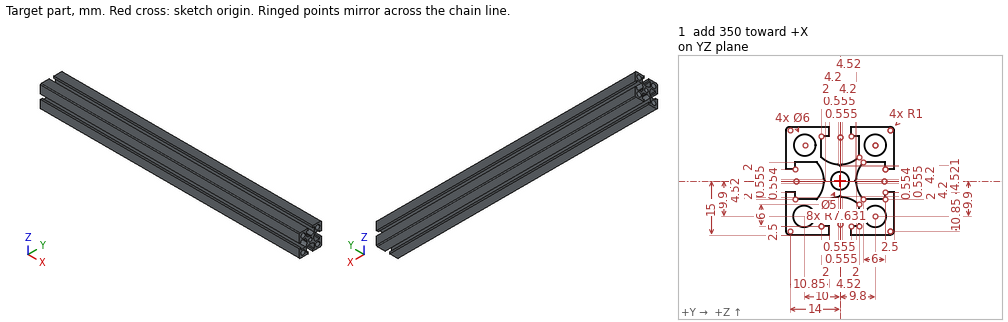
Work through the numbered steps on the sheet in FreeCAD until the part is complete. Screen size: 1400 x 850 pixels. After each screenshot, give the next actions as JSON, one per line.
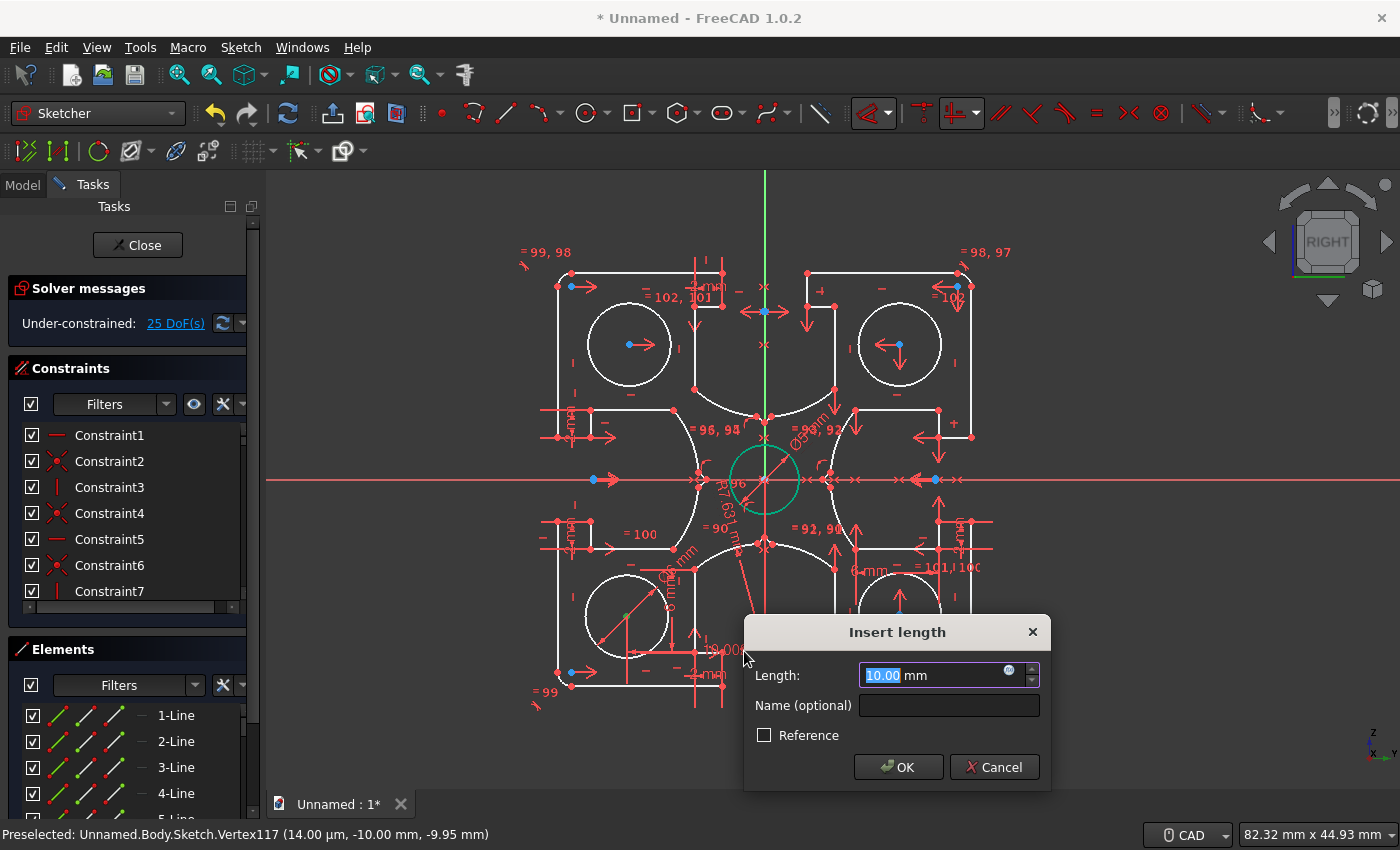
{"action": "type", "text": "10"}
{"action": "key", "text": "Return"}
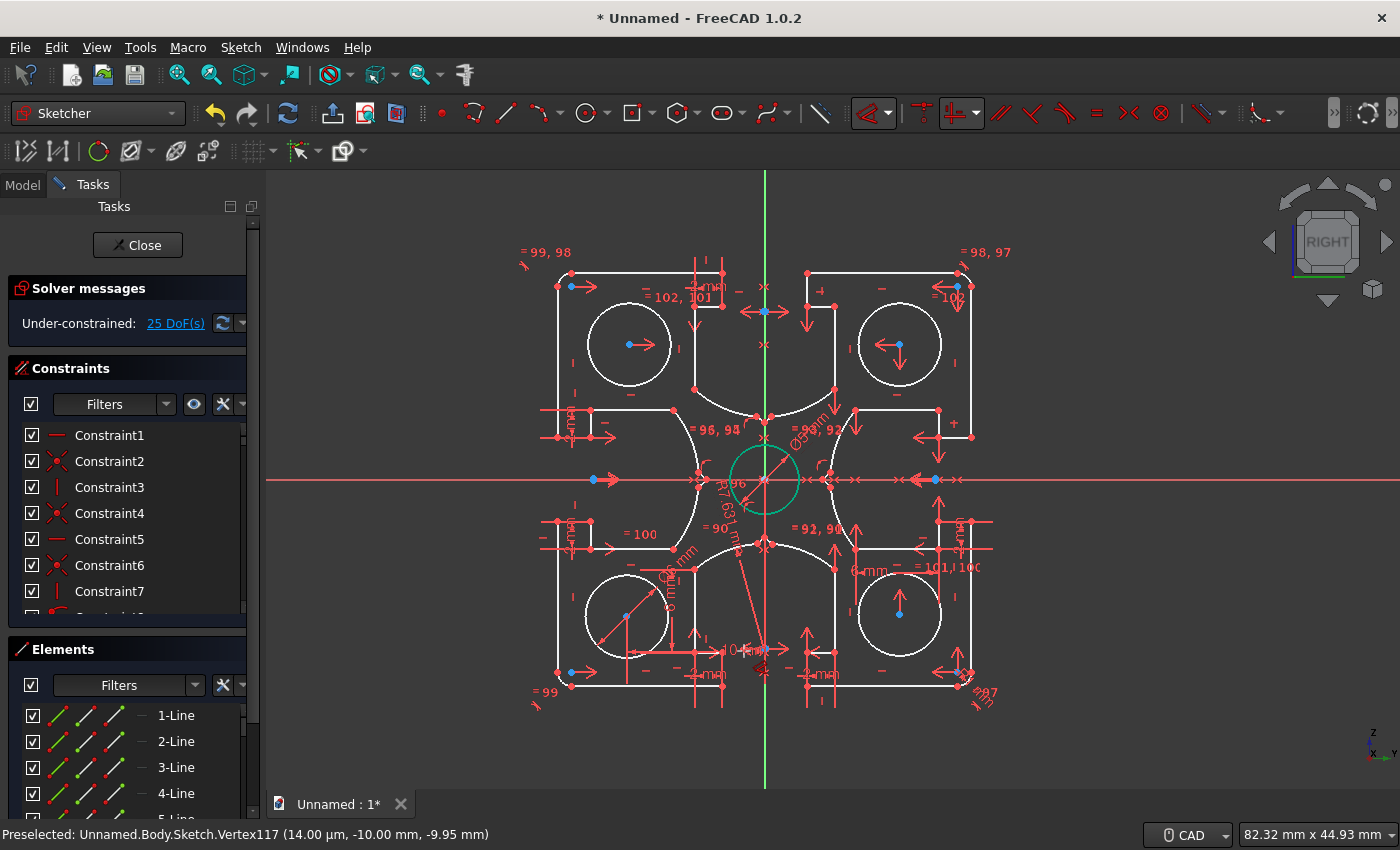
{"action": "scroll", "coordinate": [722, 676], "scroll_direction": "up", "scroll_amount": 2}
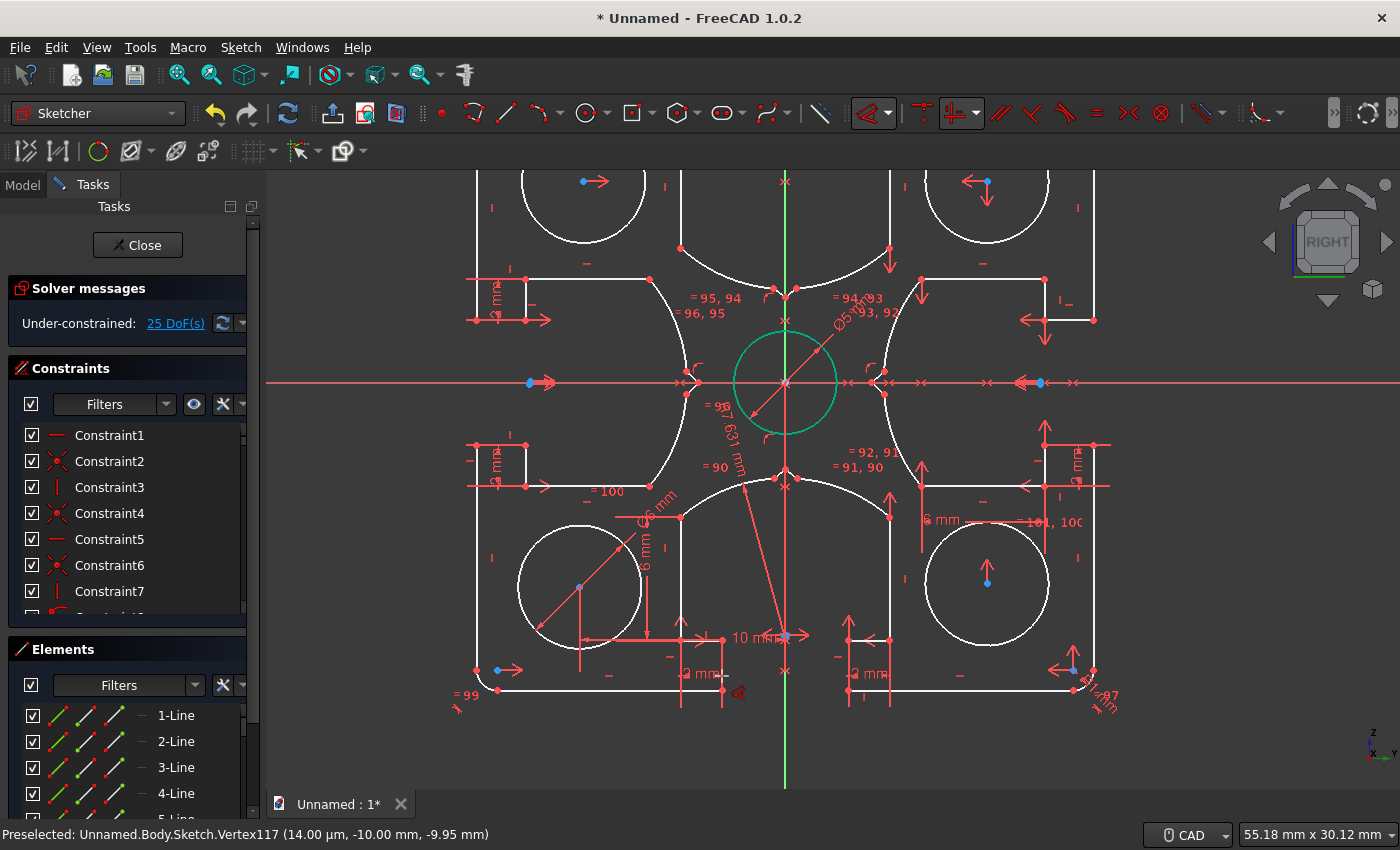
{"action": "left_click", "coordinate": [722, 676]}
{"action": "left_click", "coordinate": [664, 648]}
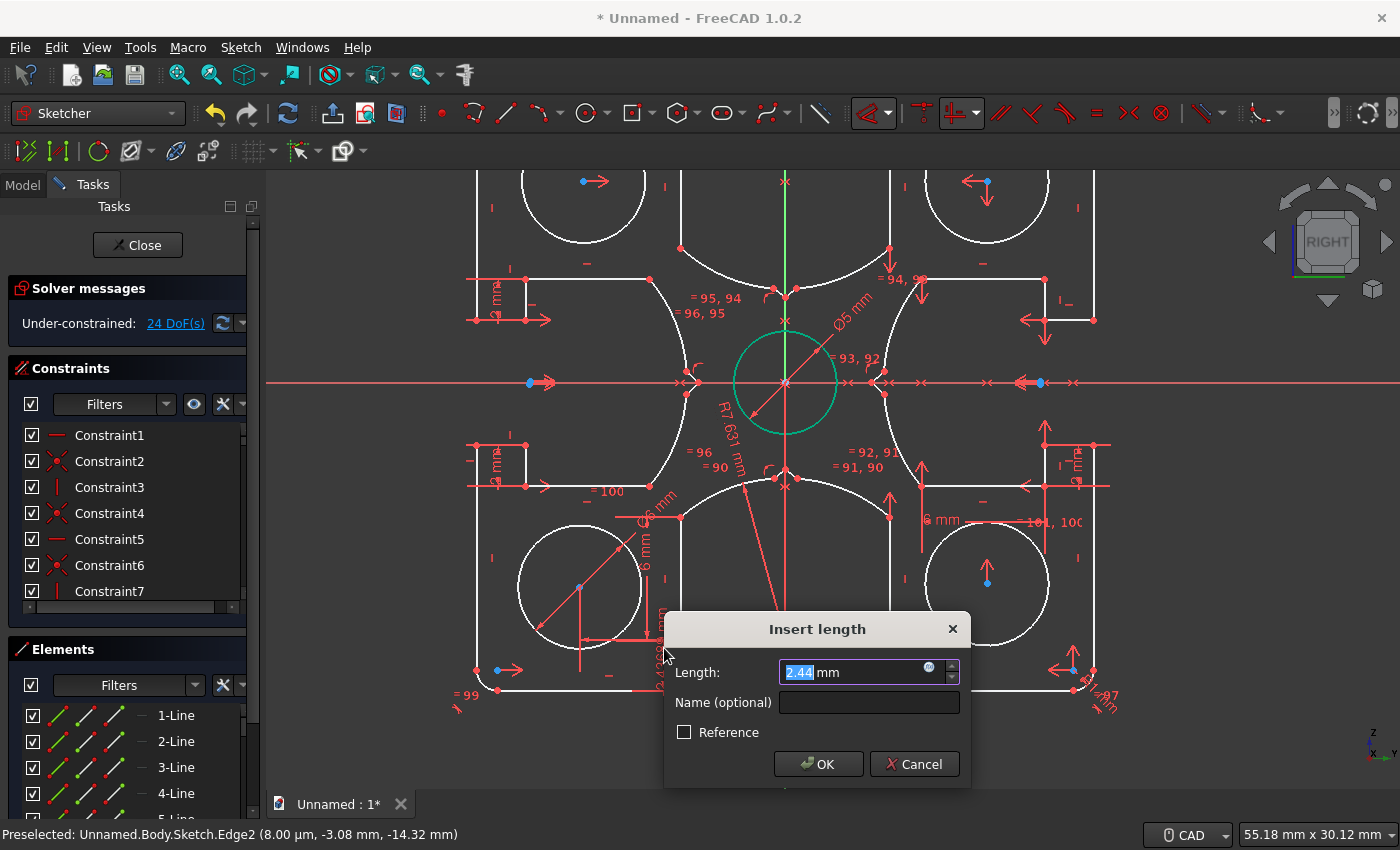
{"action": "type", "text": "2.5"}
{"action": "key", "text": "Return"}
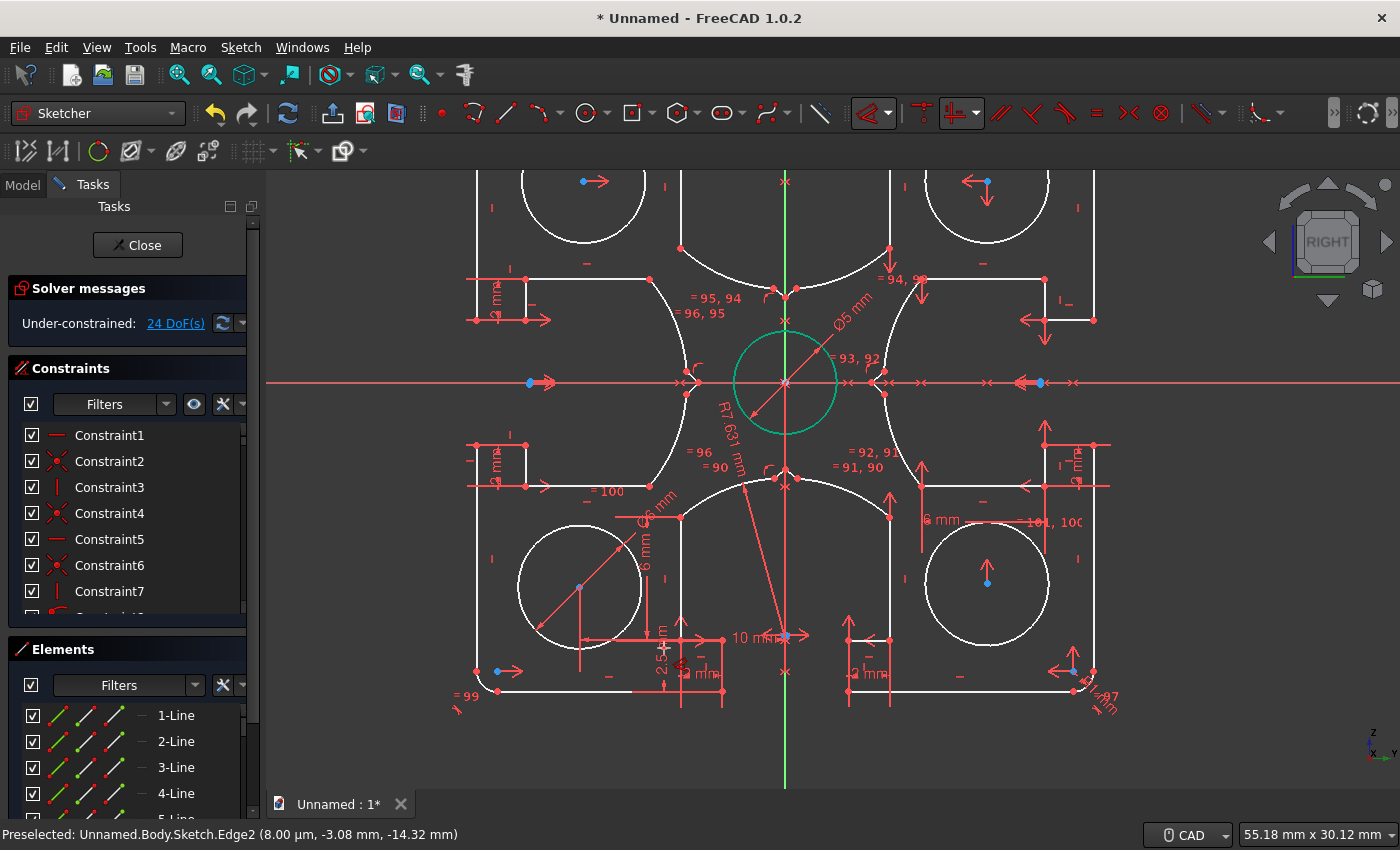
{"action": "left_click", "coordinate": [1079, 445]}
{"action": "left_click", "coordinate": [1069, 411]}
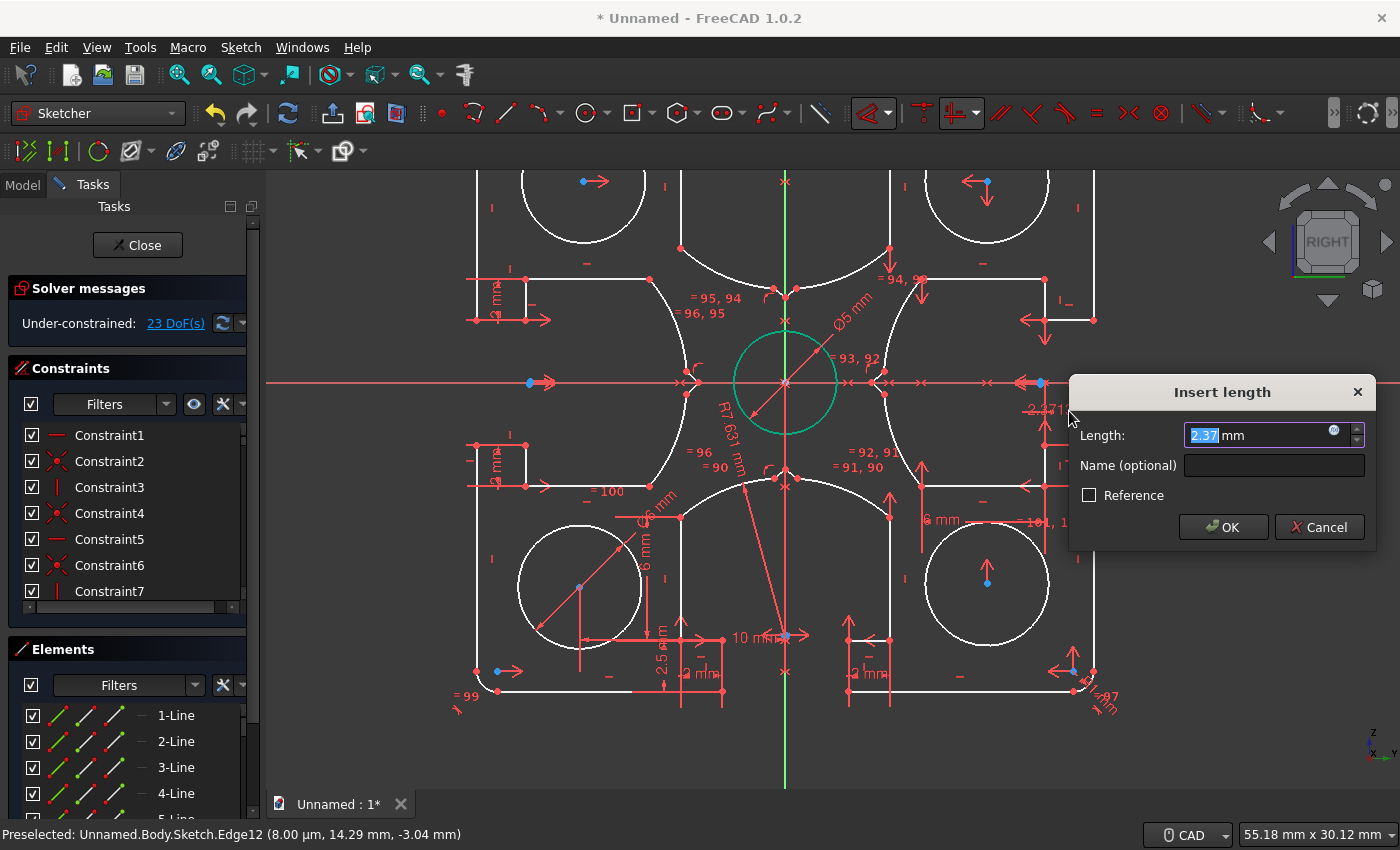
{"action": "type", "text": "2.5"}
{"action": "key", "text": "Return"}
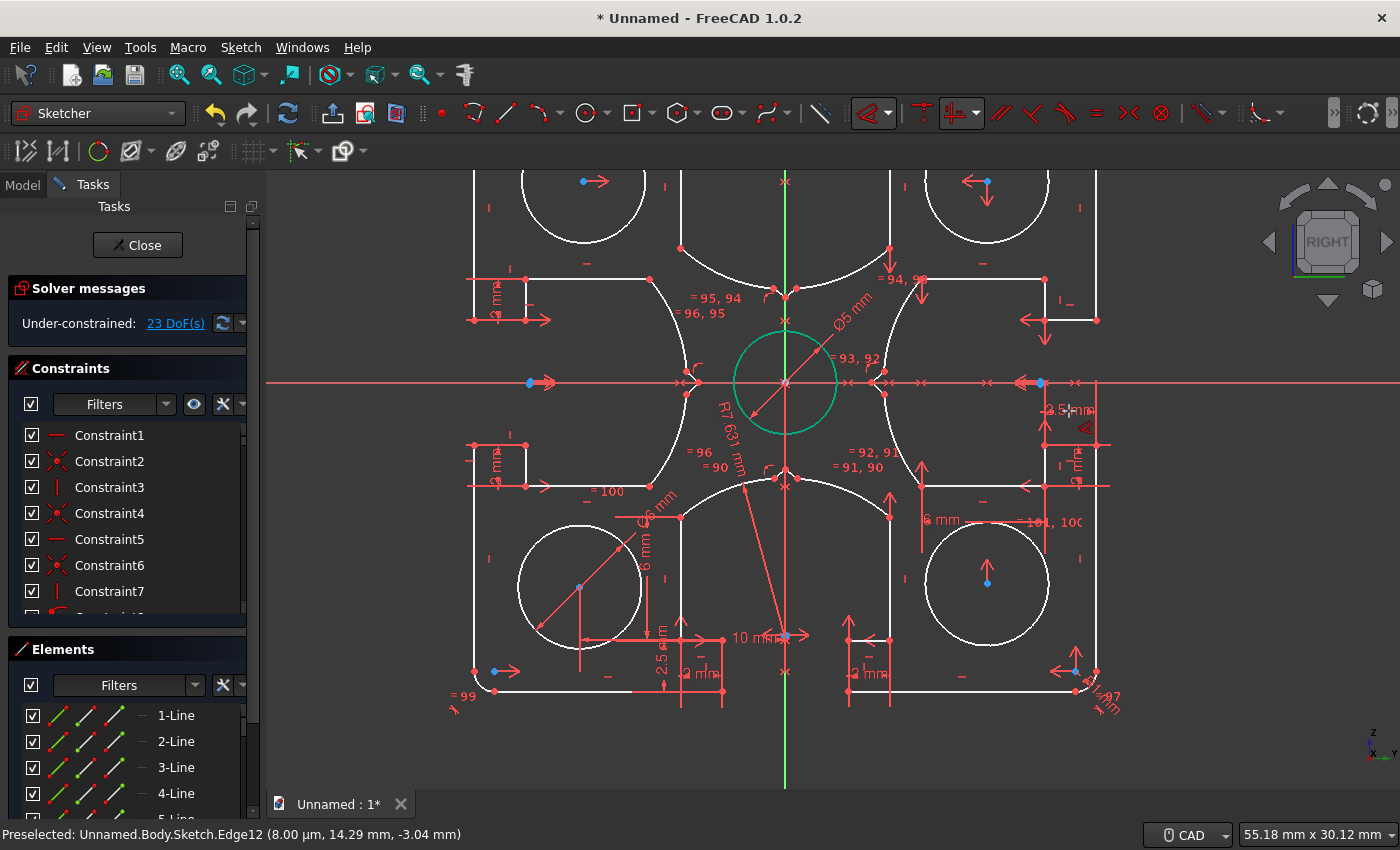
{"action": "left_click", "coordinate": [495, 692]}
{"action": "left_click", "coordinate": [640, 726]}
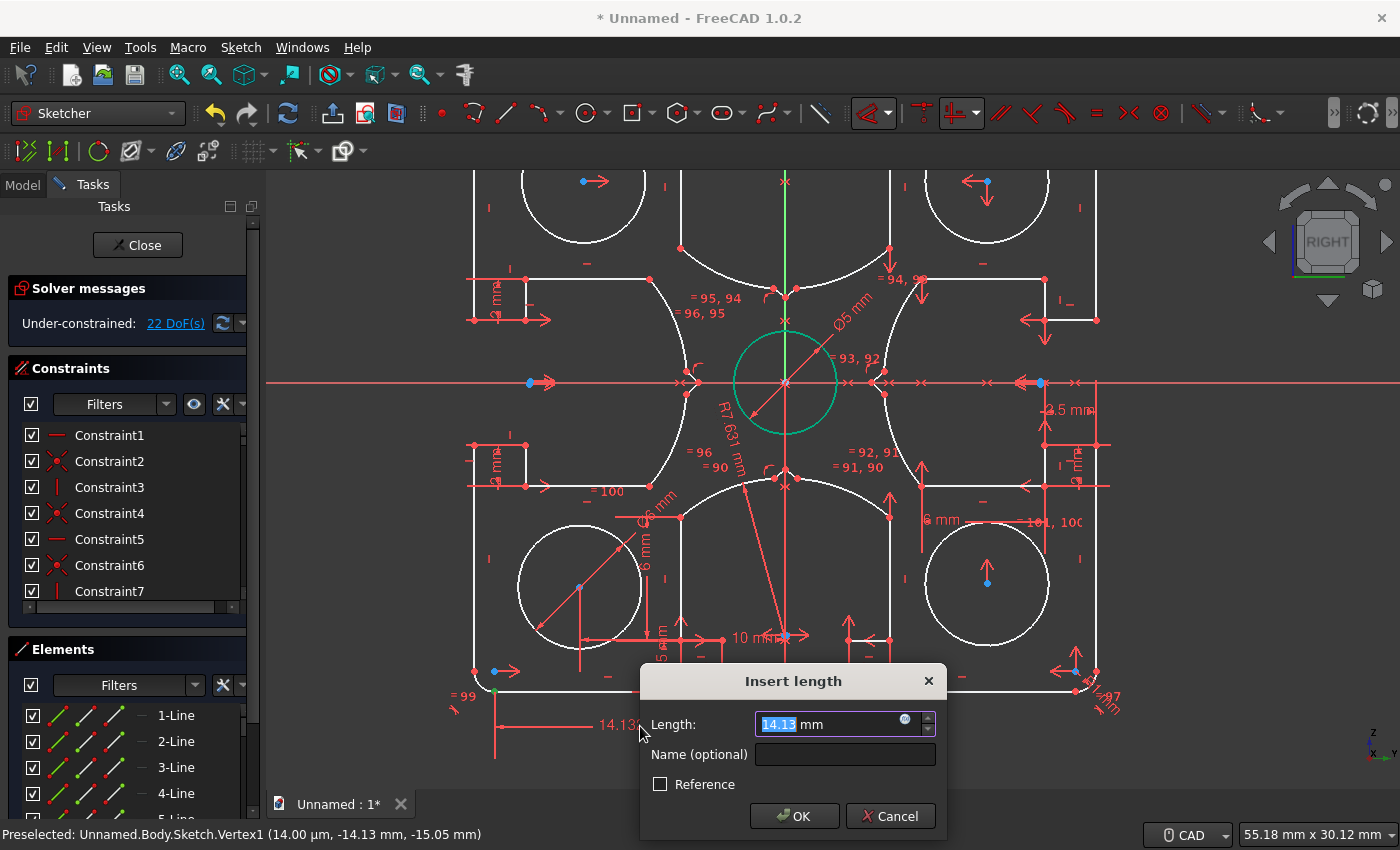
{"action": "type", "text": "14"}
{"action": "key", "text": "Return"}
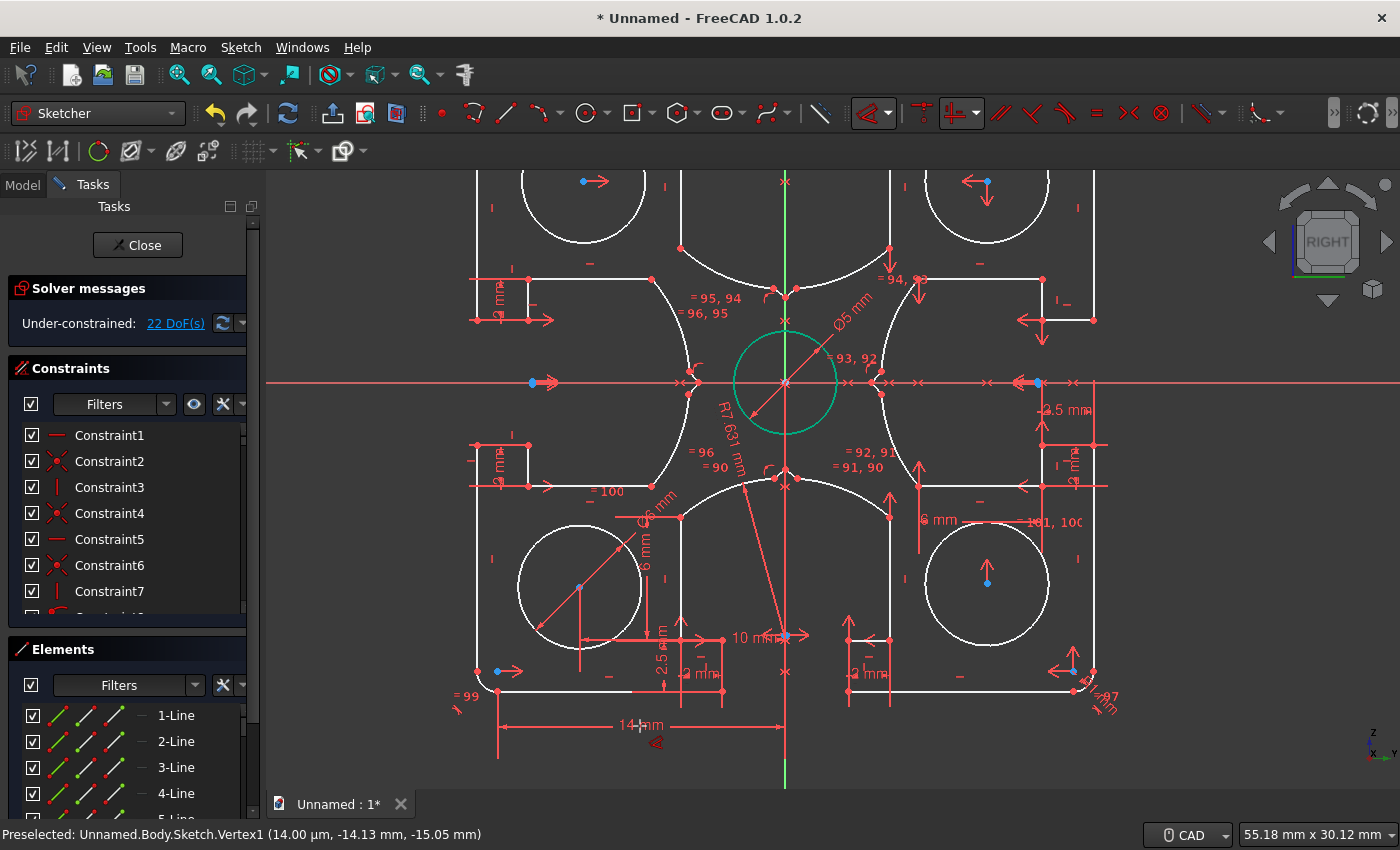
{"action": "left_click", "coordinate": [498, 692]}
{"action": "left_click", "coordinate": [464, 537]}